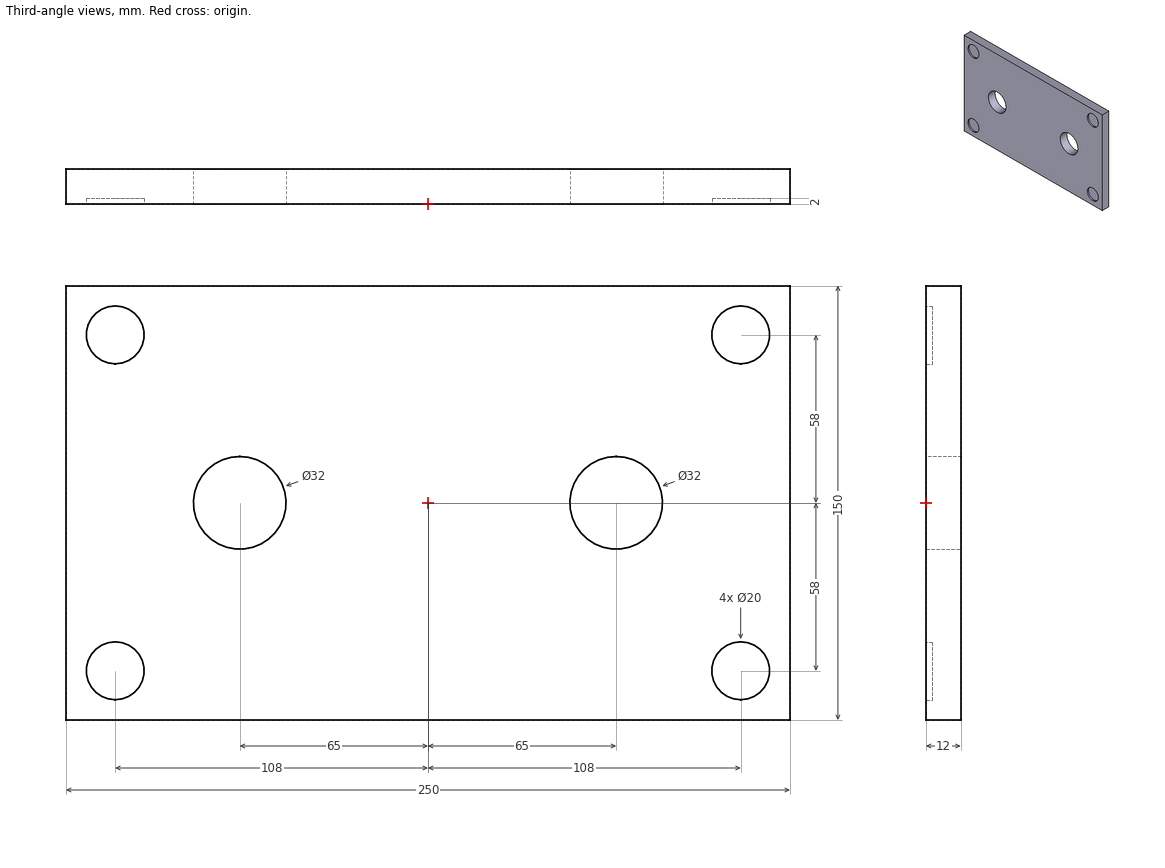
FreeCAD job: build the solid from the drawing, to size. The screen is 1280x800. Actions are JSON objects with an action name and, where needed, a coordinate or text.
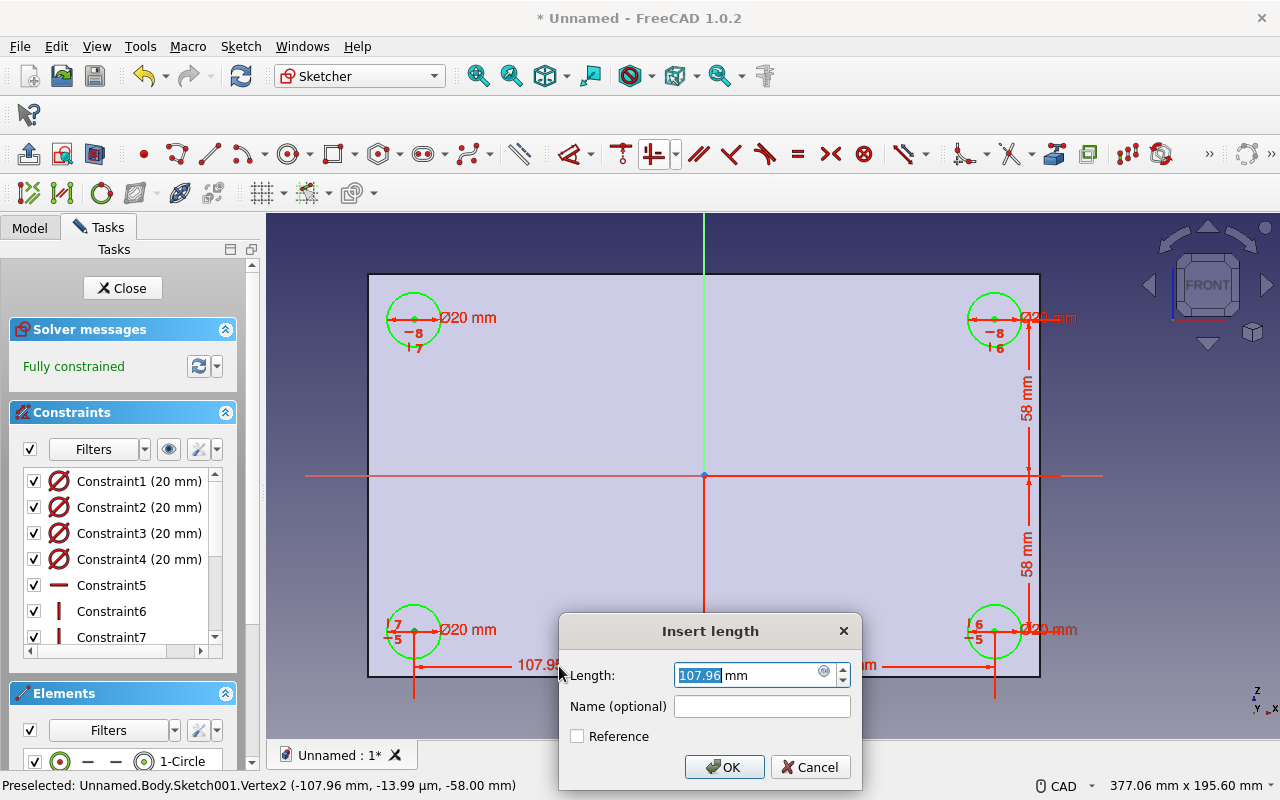
{"action": "type", "text": "108"}
{"action": "key", "text": "Return"}
{"action": "key", "text": "Escape"}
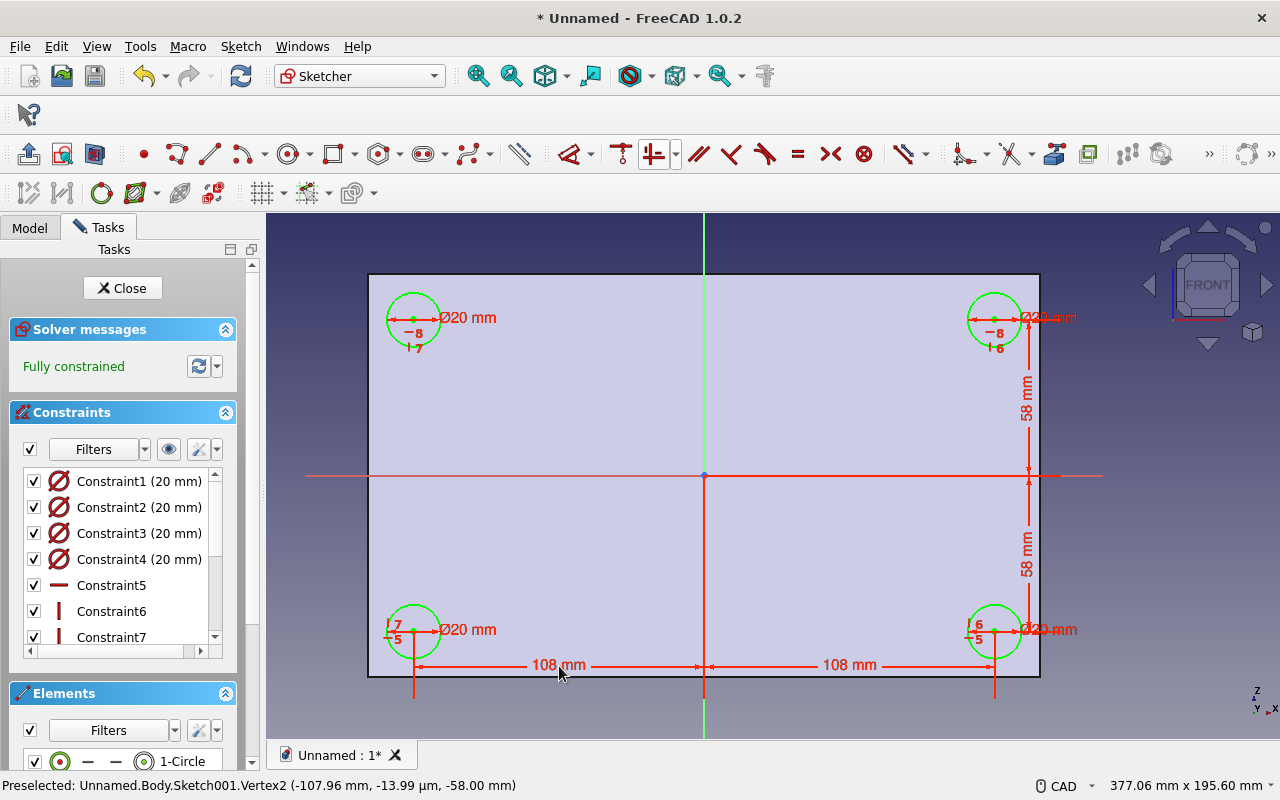
{"action": "left_click", "coordinate": [123, 288]}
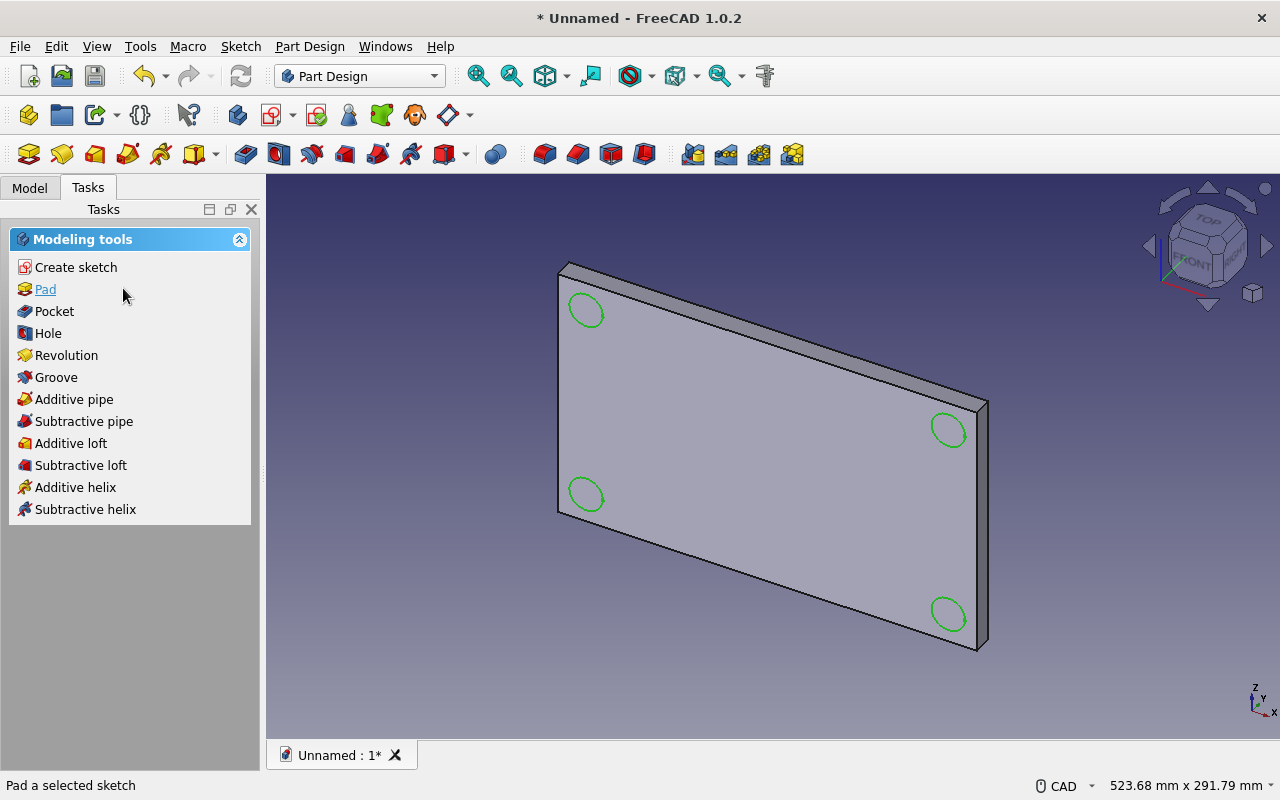
{"action": "left_click", "coordinate": [246, 154]}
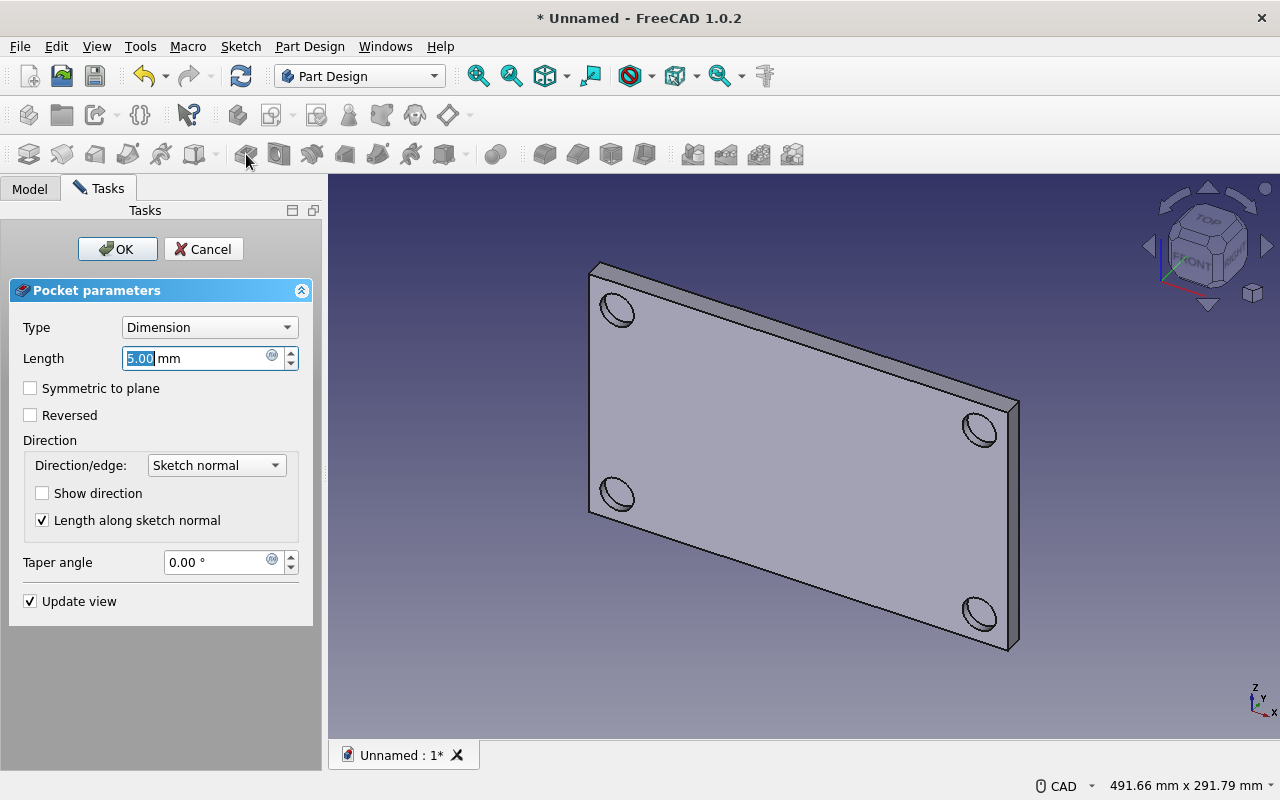
{"action": "type", "text": "2"}
{"action": "key", "text": "Tab"}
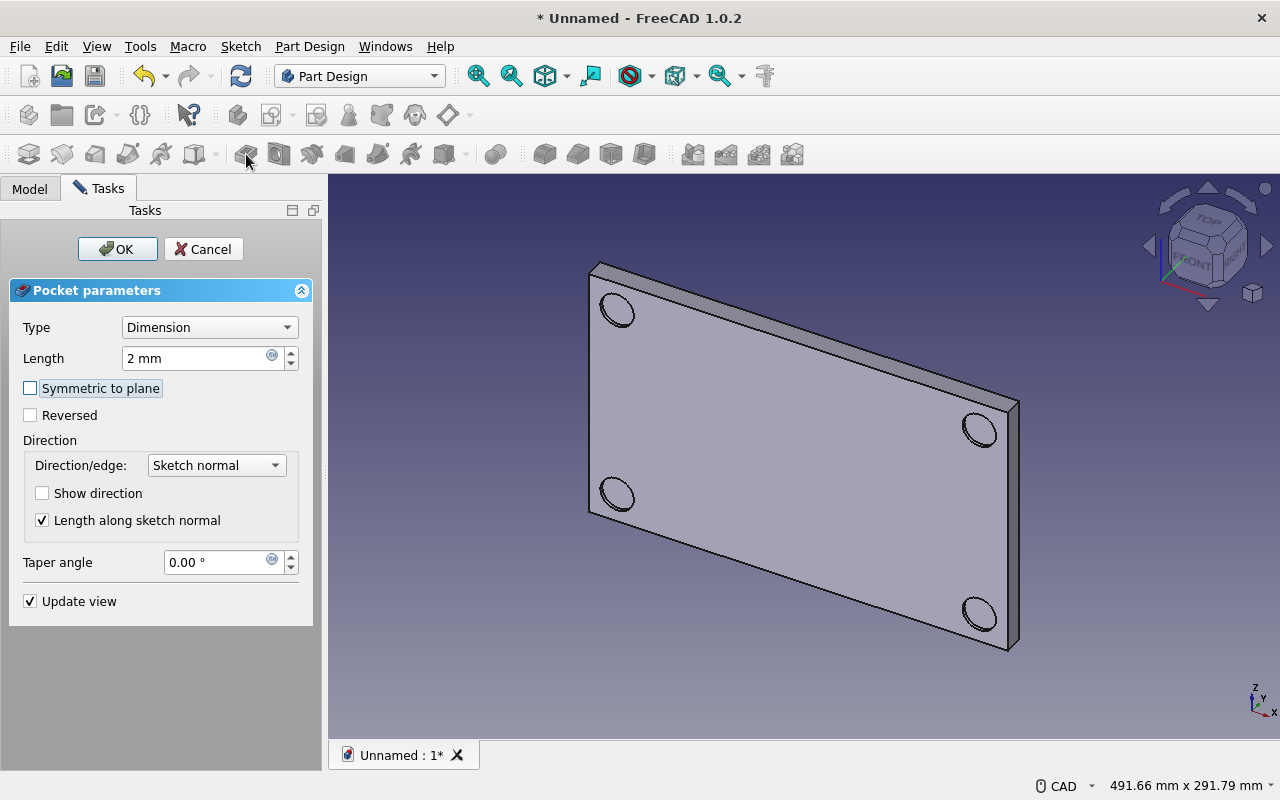
{"action": "left_click", "coordinate": [118, 249]}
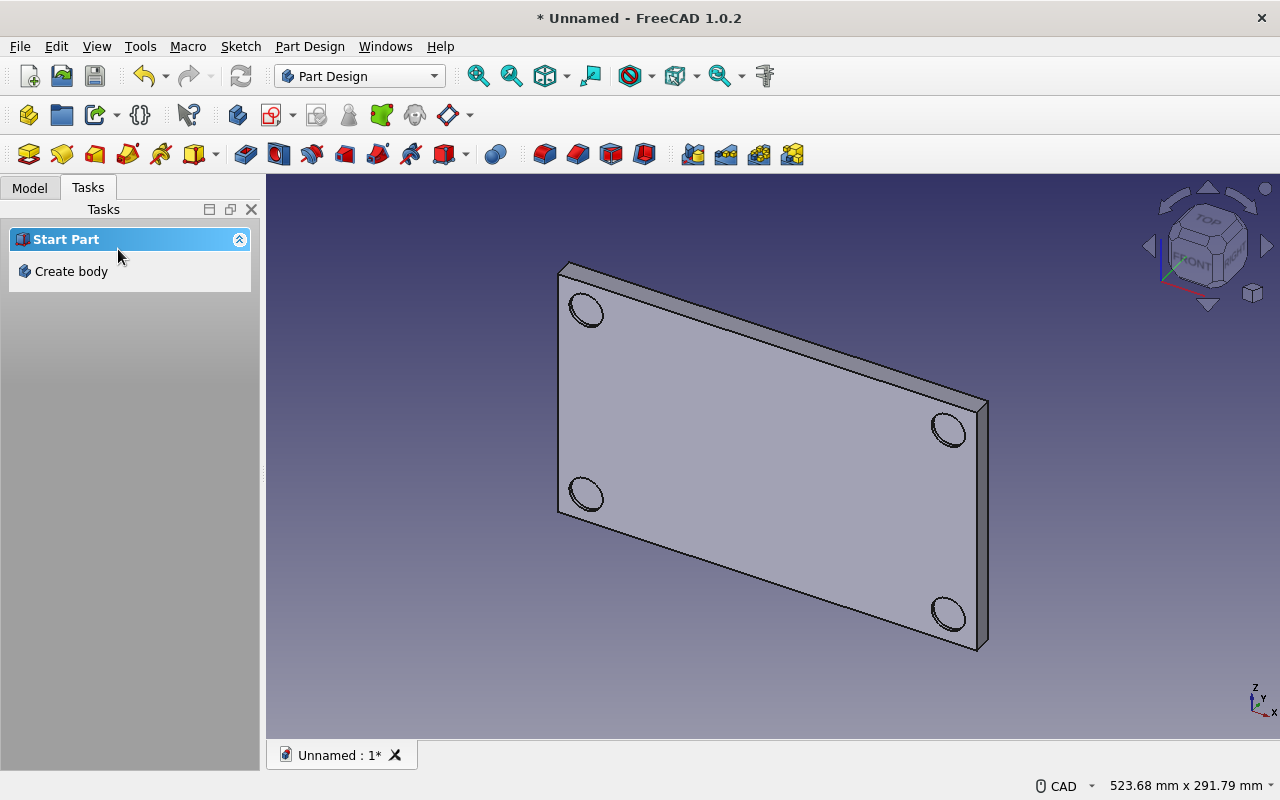
{"action": "key", "text": "4"}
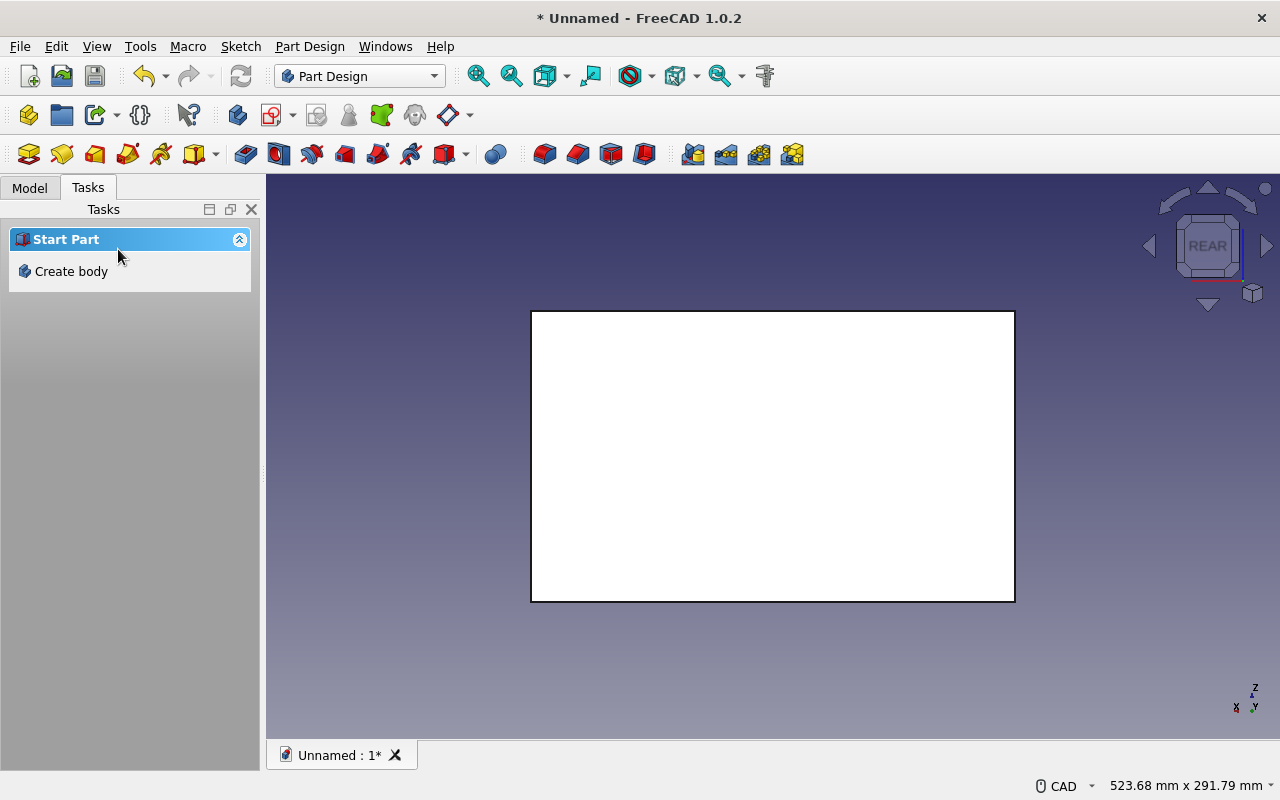
{"action": "left_click", "coordinate": [704, 455]}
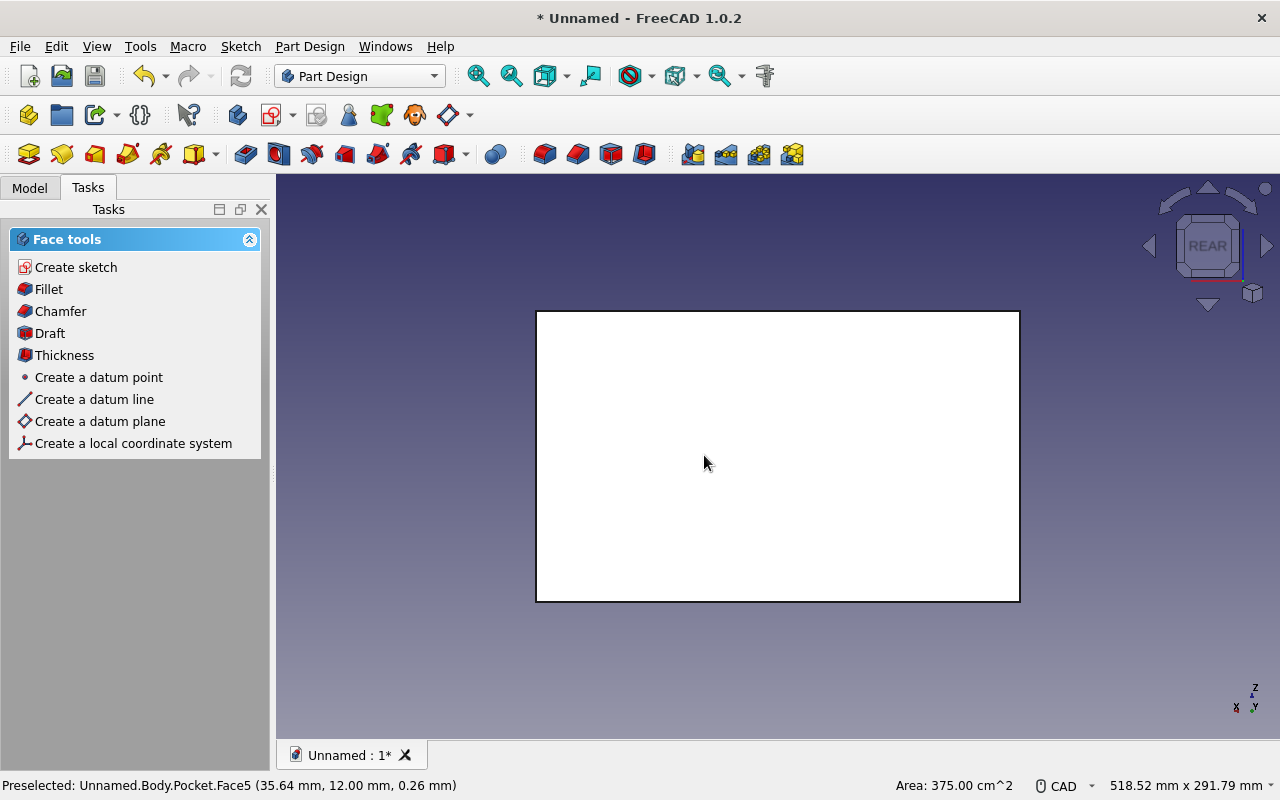
{"action": "left_click", "coordinate": [270, 116]}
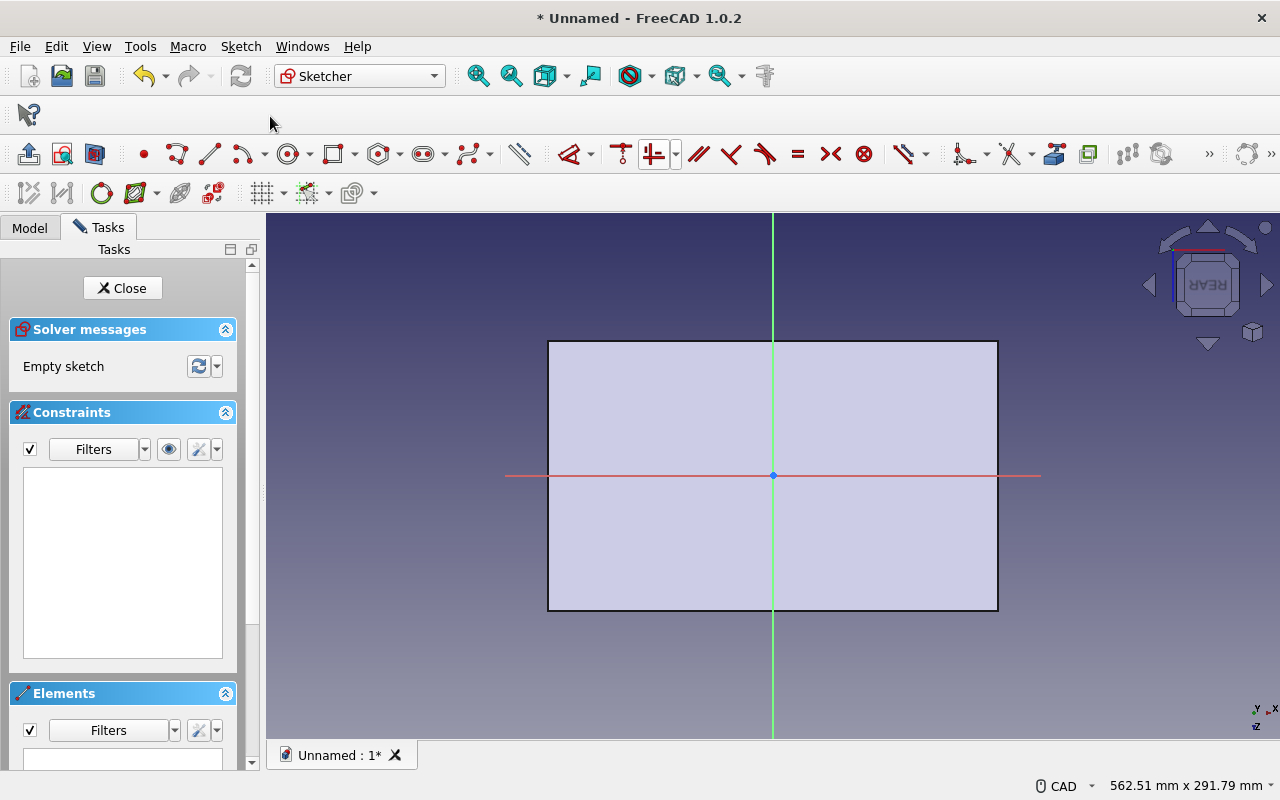
{"action": "scroll", "coordinate": [646, 476], "scroll_direction": "up", "scroll_amount": 9}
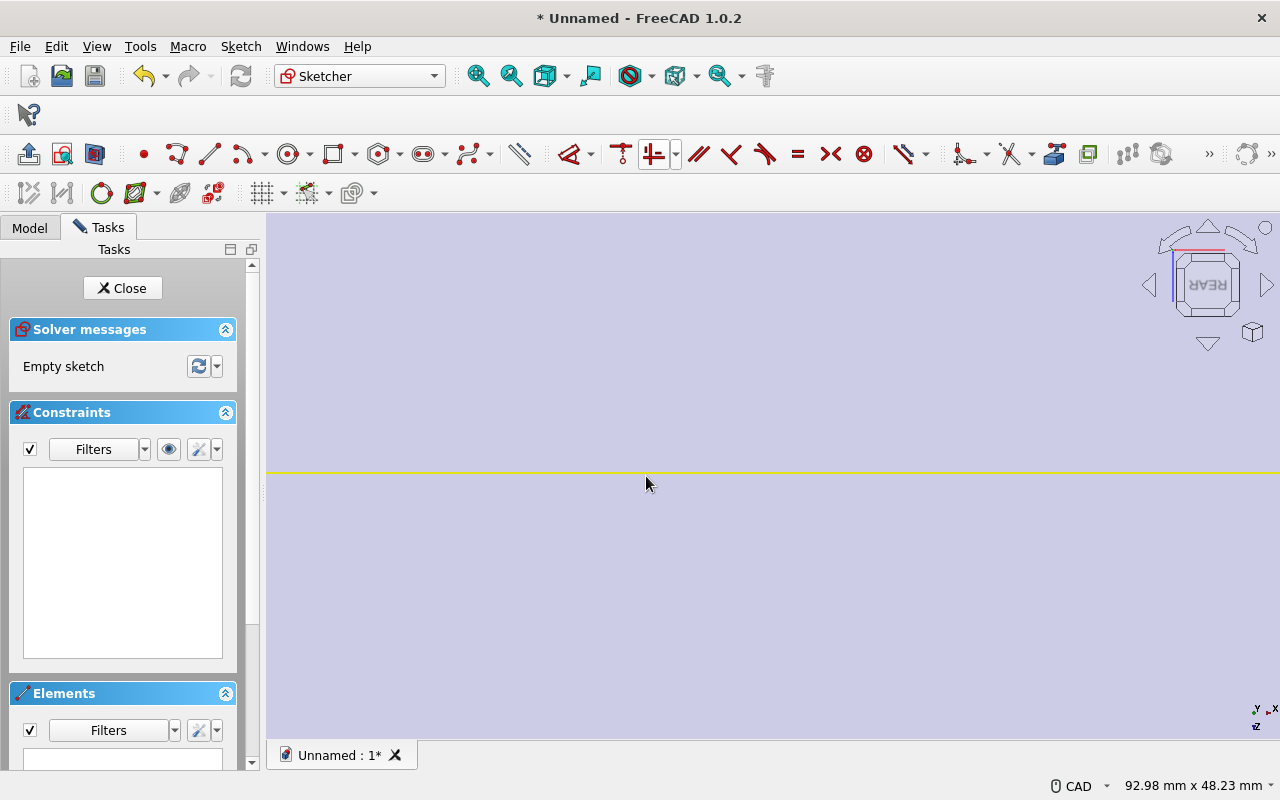
{"action": "key", "text": "g c"}